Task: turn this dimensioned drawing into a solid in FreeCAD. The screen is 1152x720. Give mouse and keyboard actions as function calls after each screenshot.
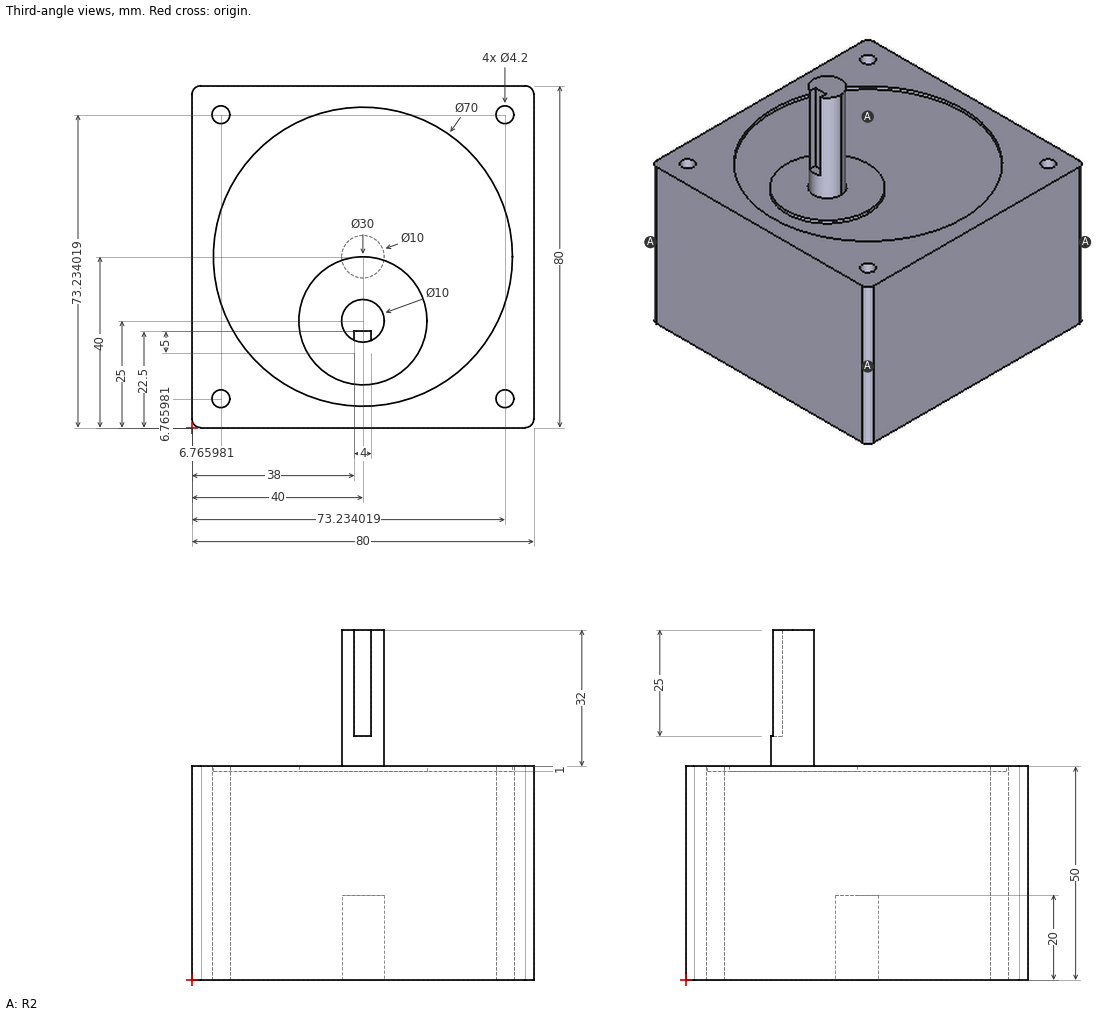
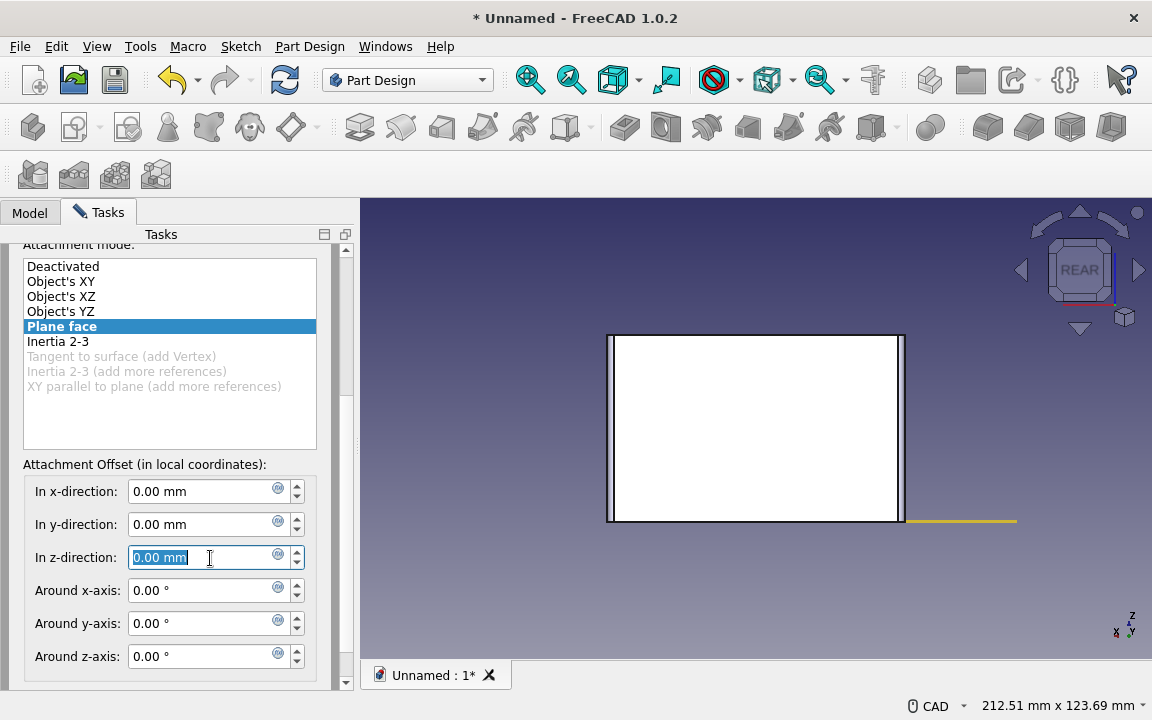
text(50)
key(Tab)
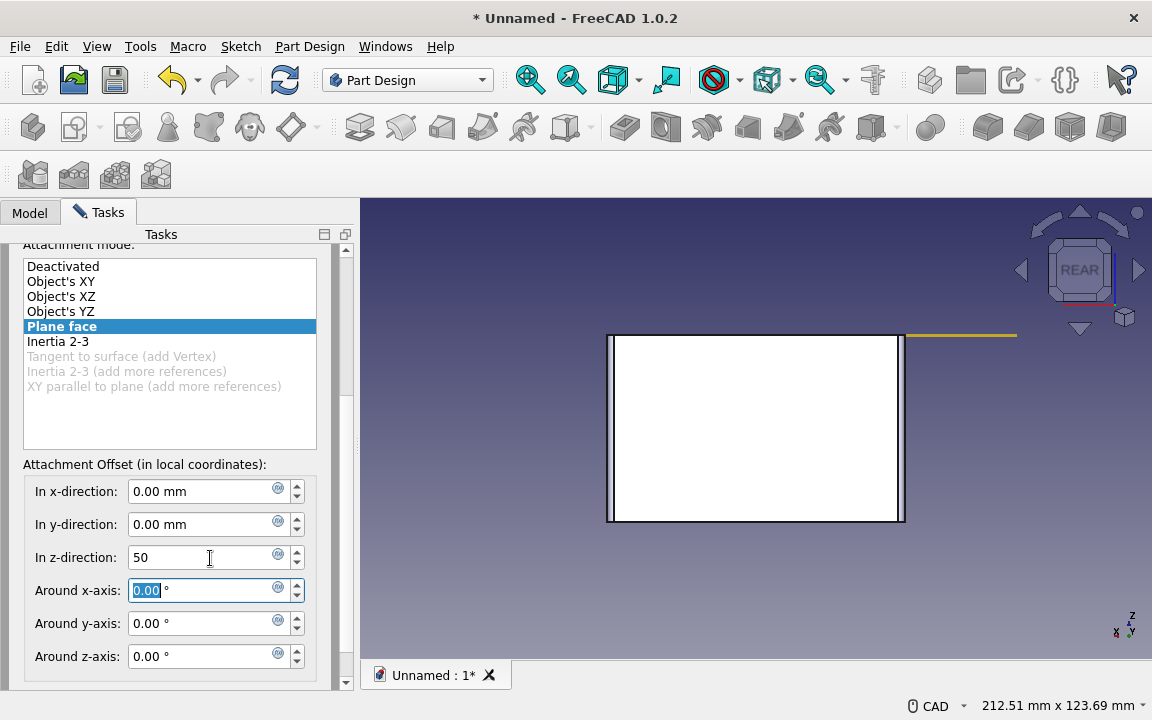
scroll(346, 467, up, 5)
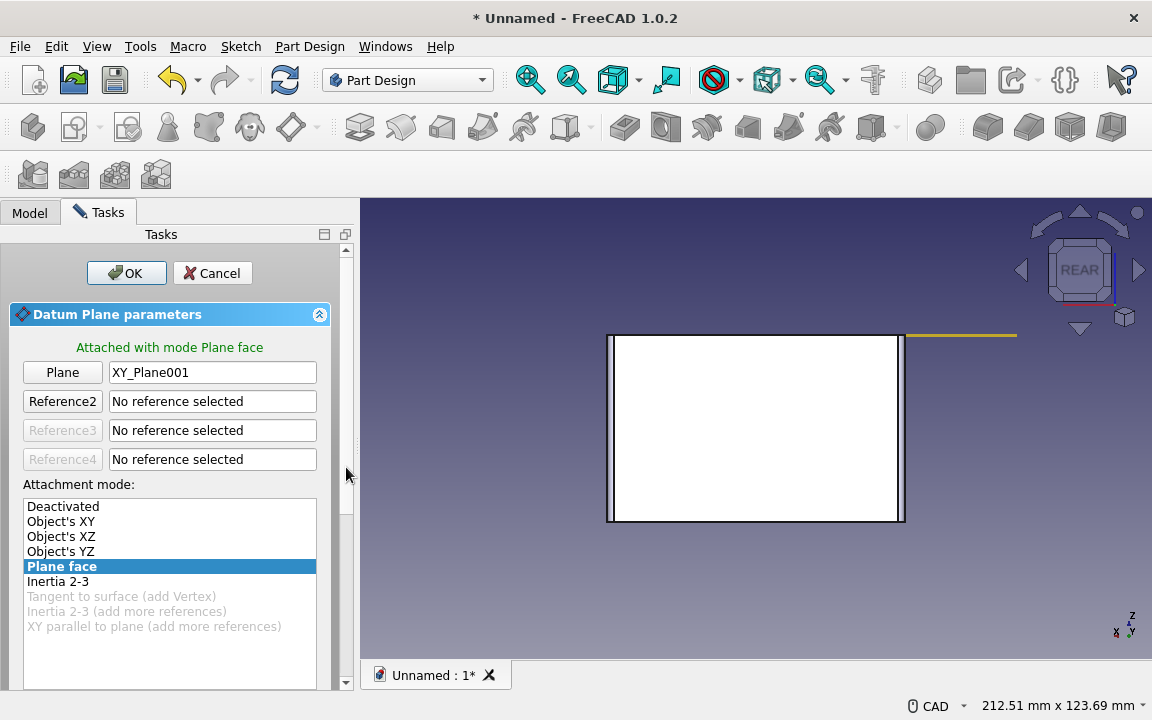
click(127, 273)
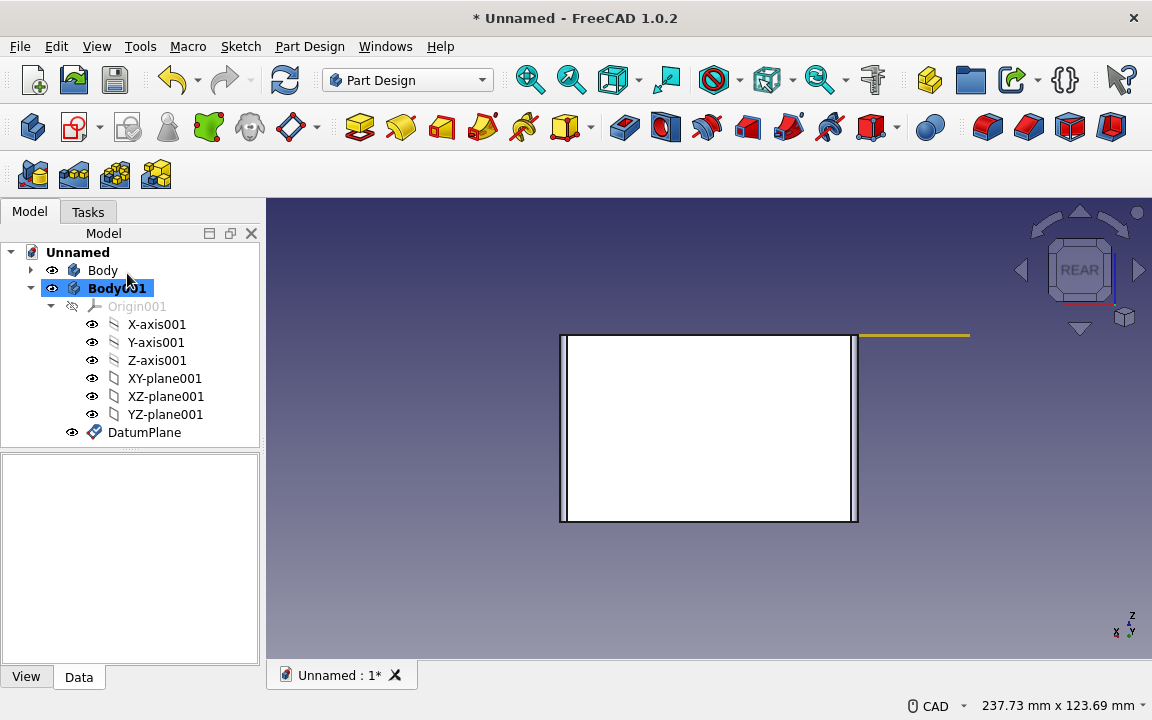
click(117, 432)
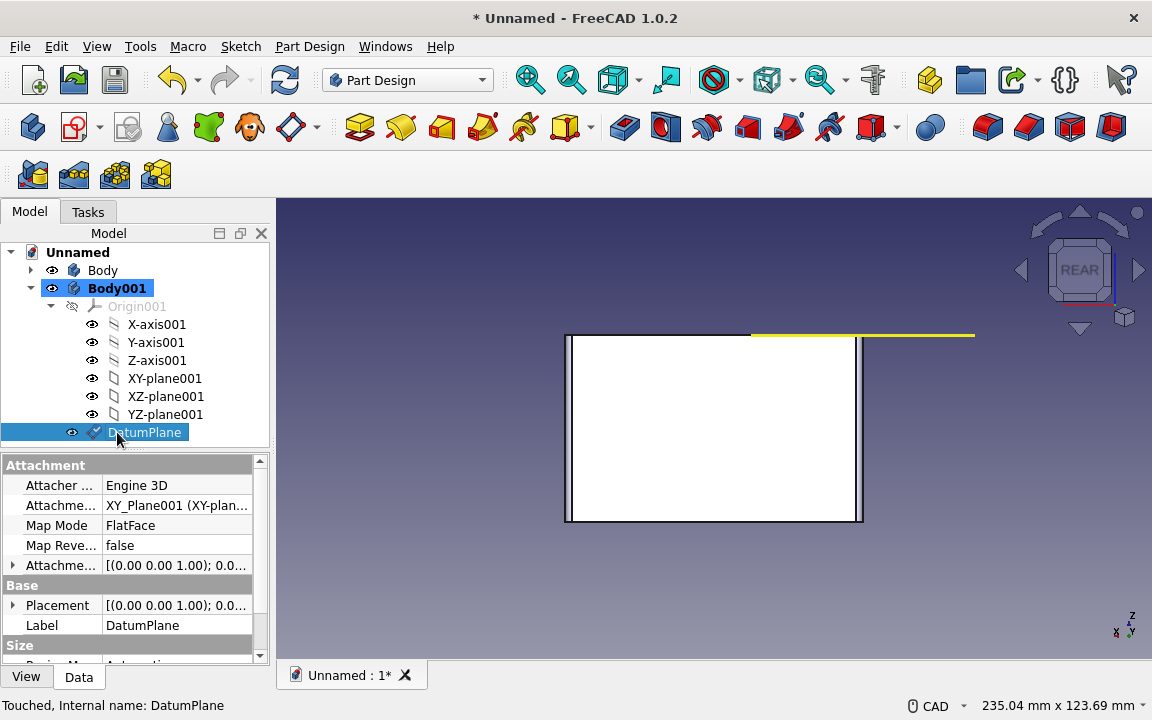
click(74, 128)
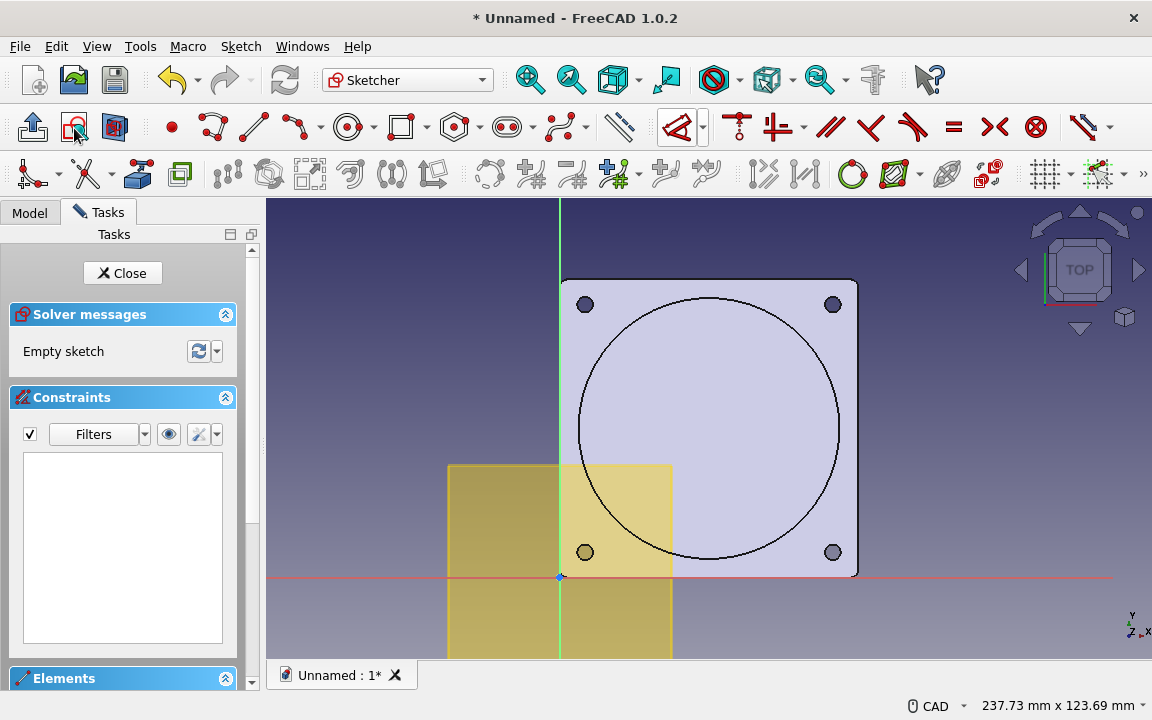
scroll(720, 493, up, 10)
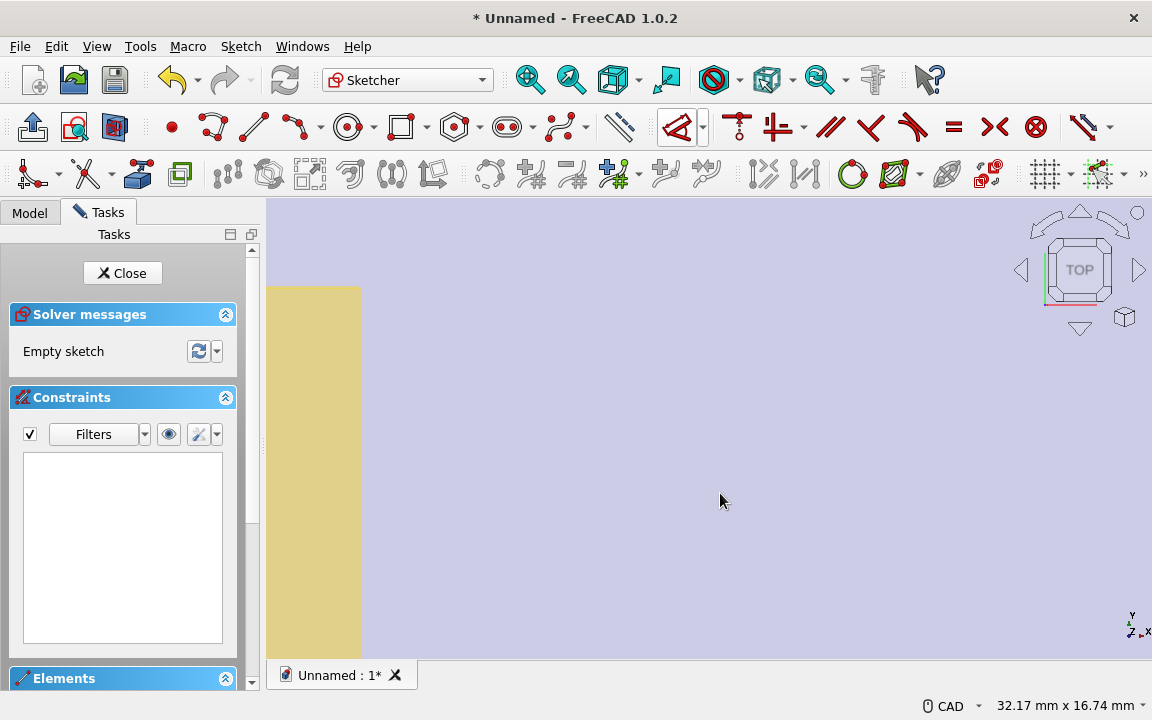
click(348, 128)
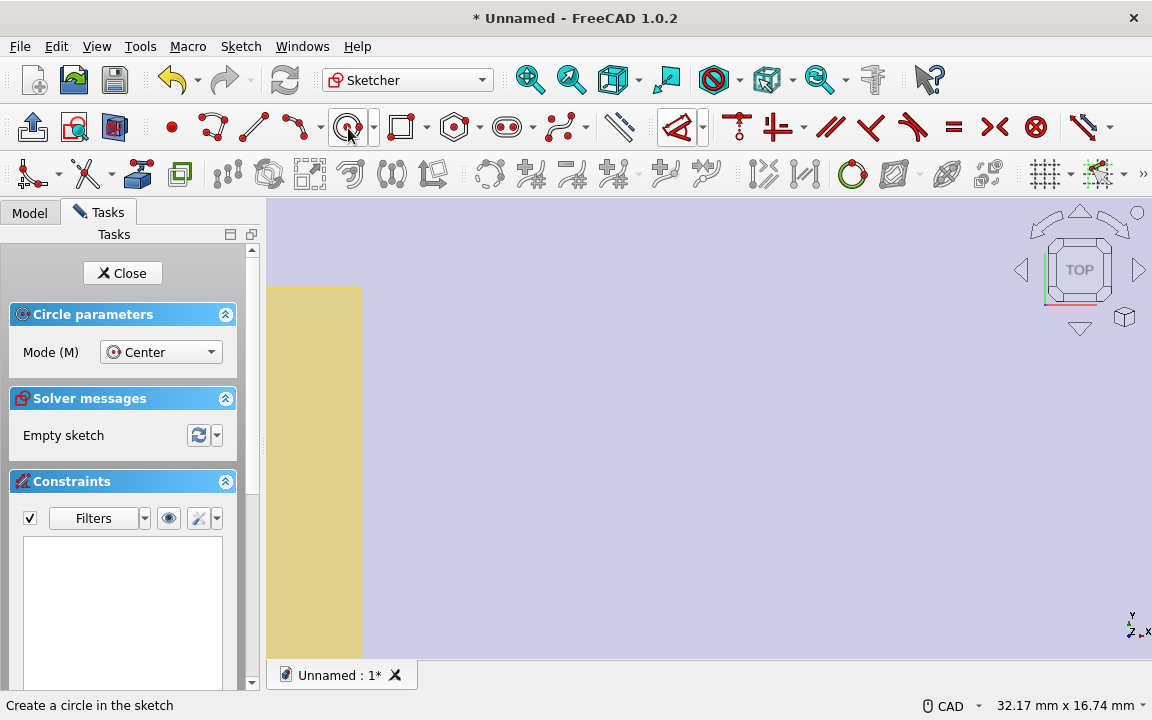
click(635, 425)
click(733, 328)
key(Escape)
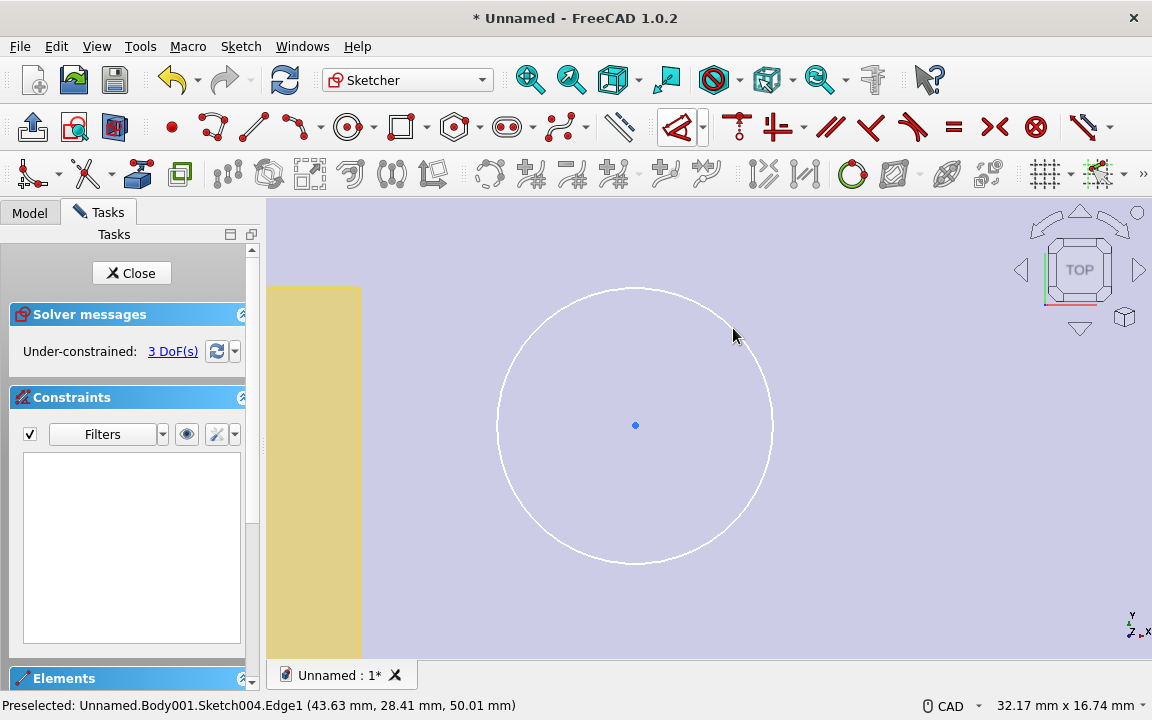
click(732, 328)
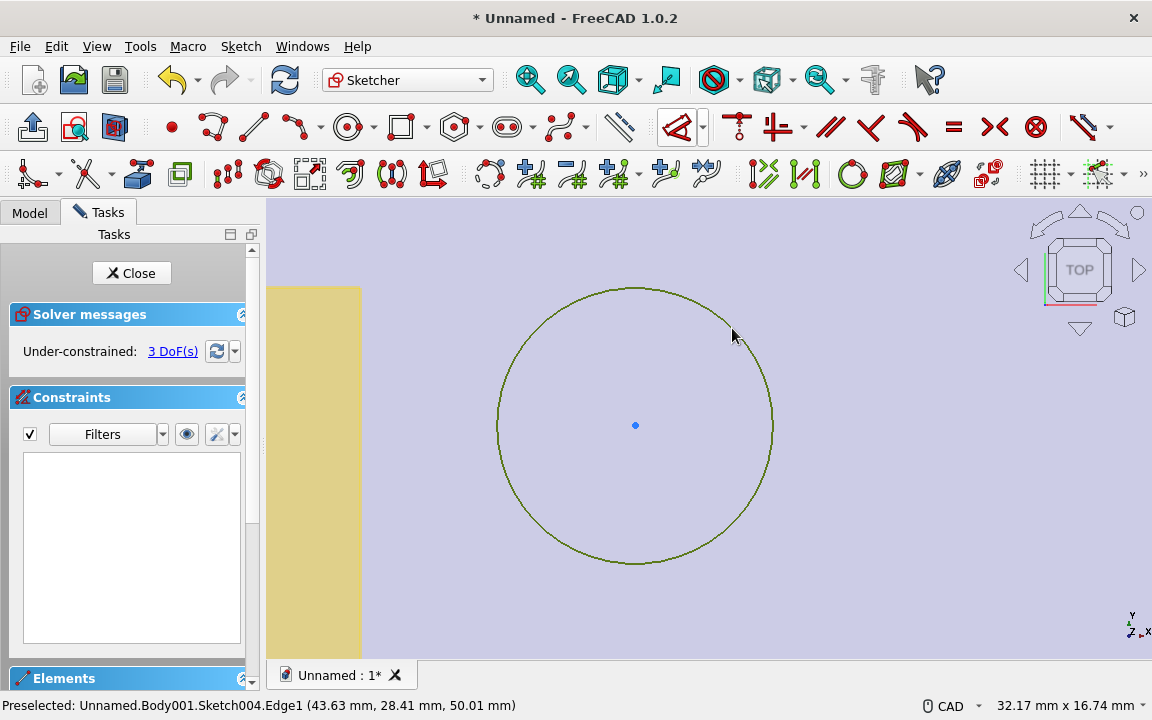
key(k)
key(o)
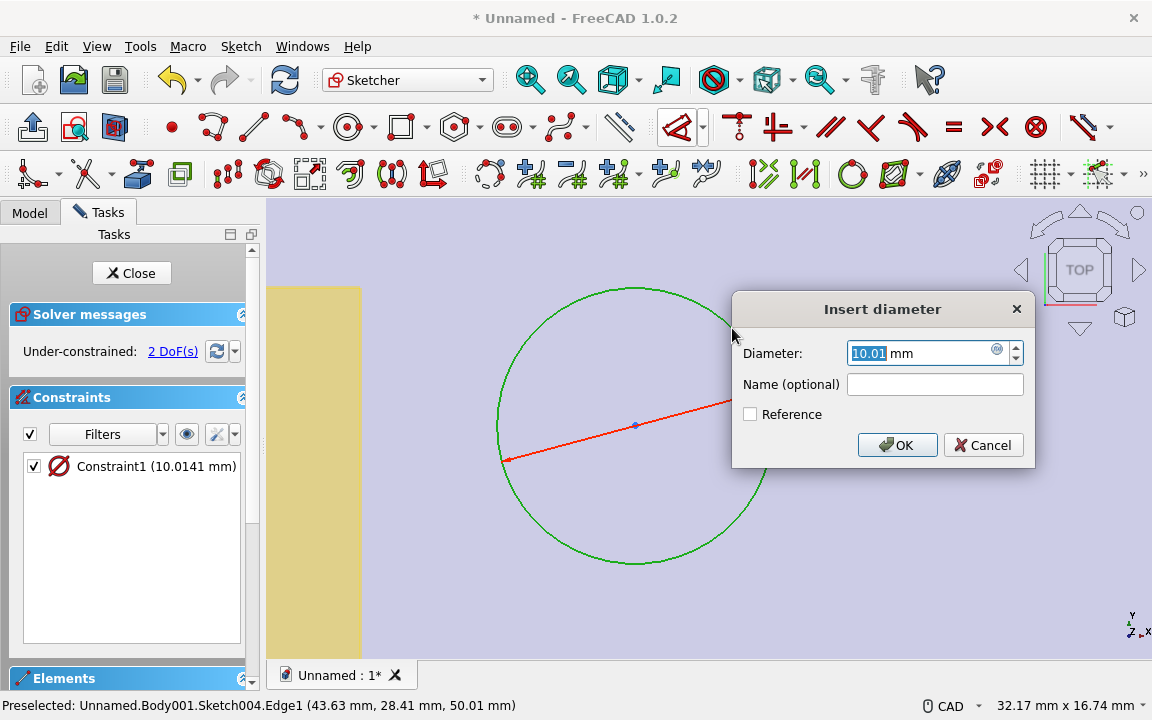
text(10)
key(Return)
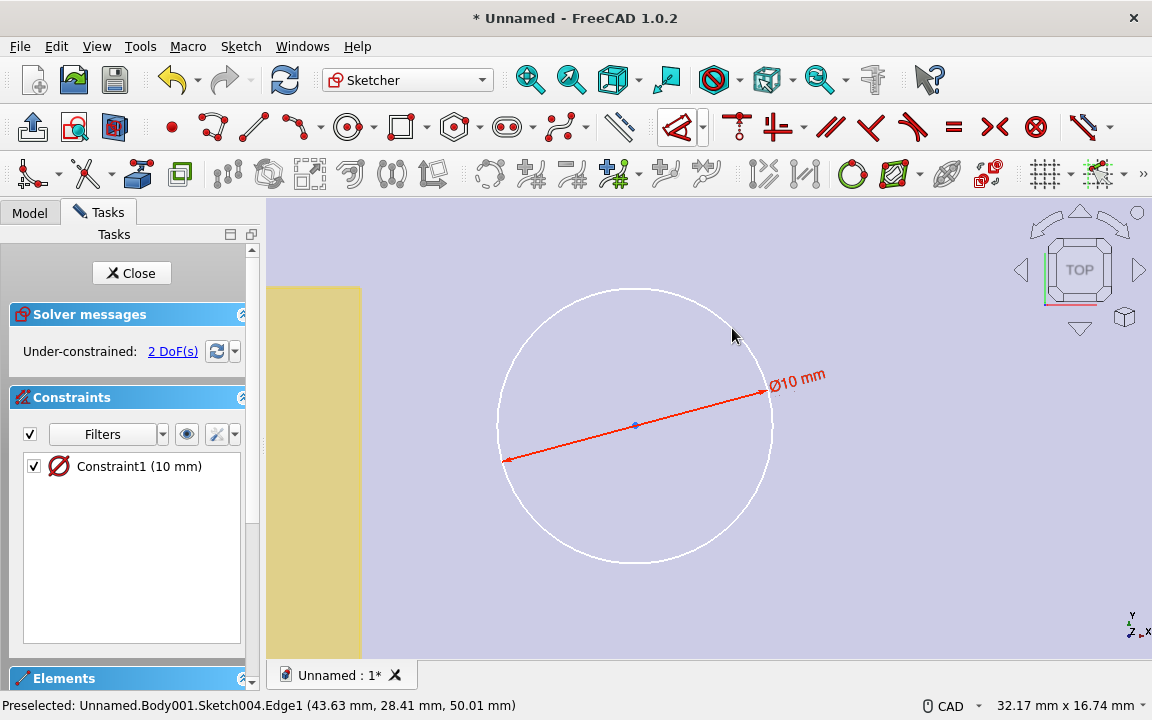
click(635, 426)